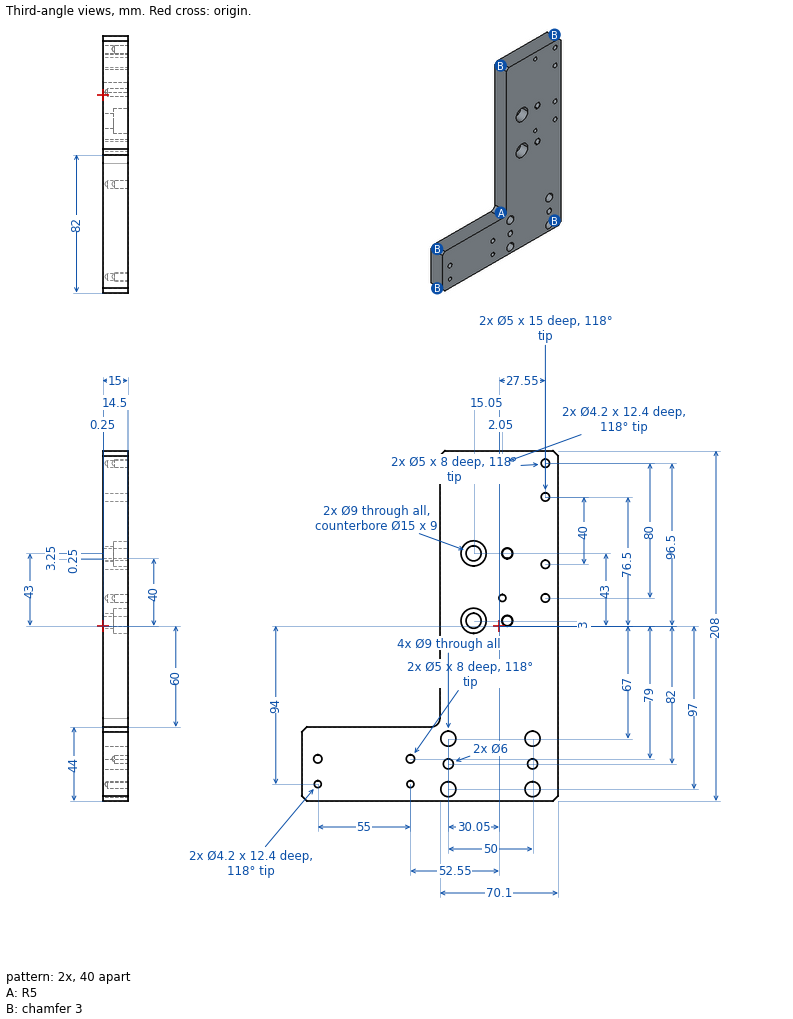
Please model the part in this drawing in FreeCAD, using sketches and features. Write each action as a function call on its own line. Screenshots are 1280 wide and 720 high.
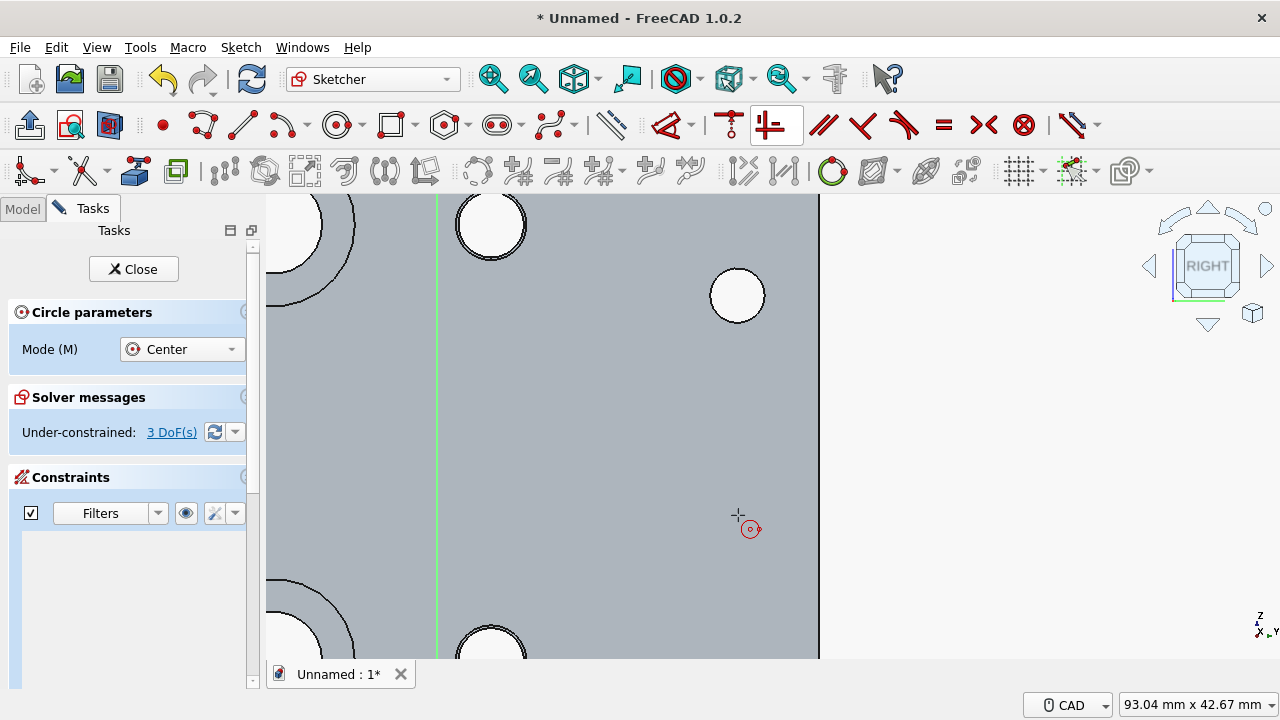
scroll(738, 516, down, 7)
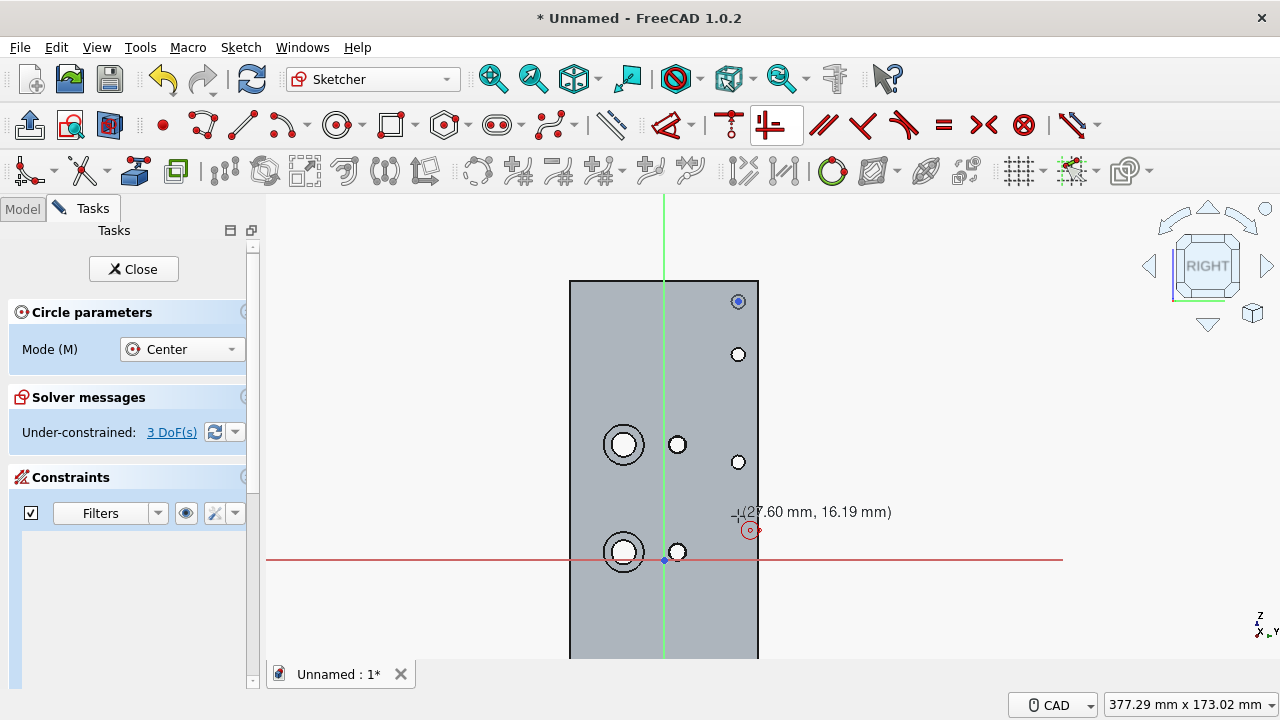
click(738, 516)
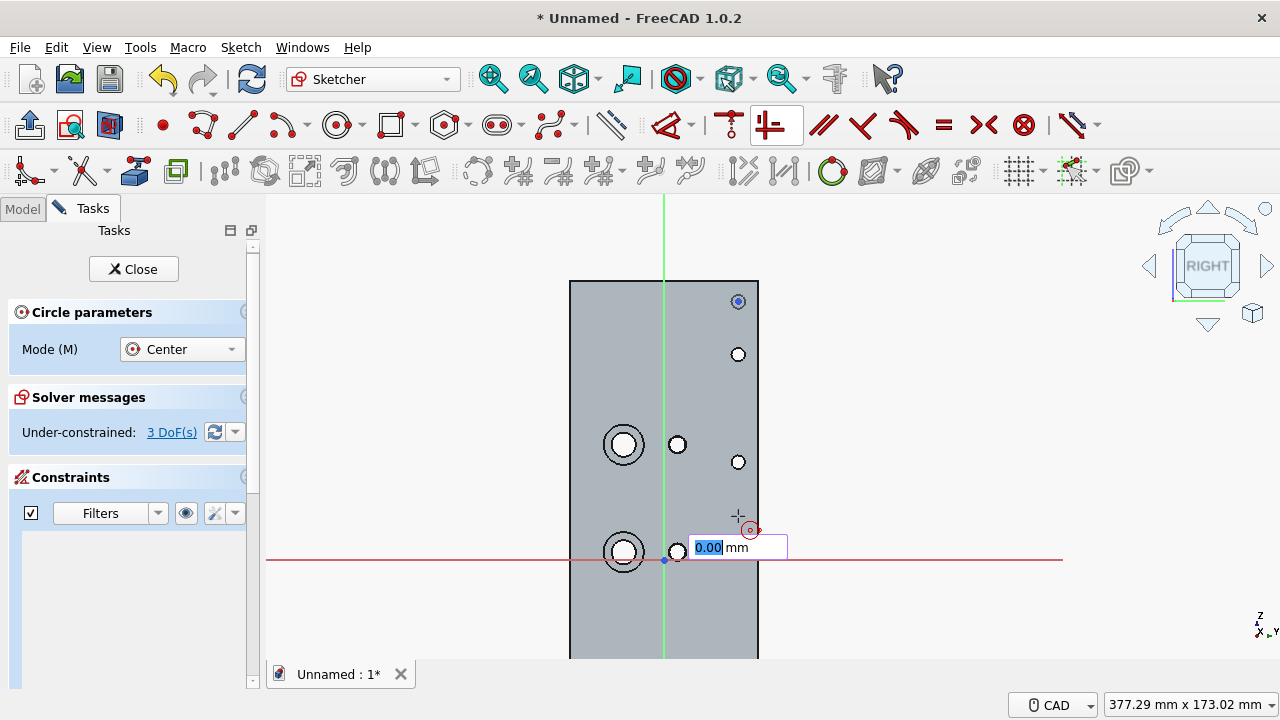
scroll(743, 511, up, 5)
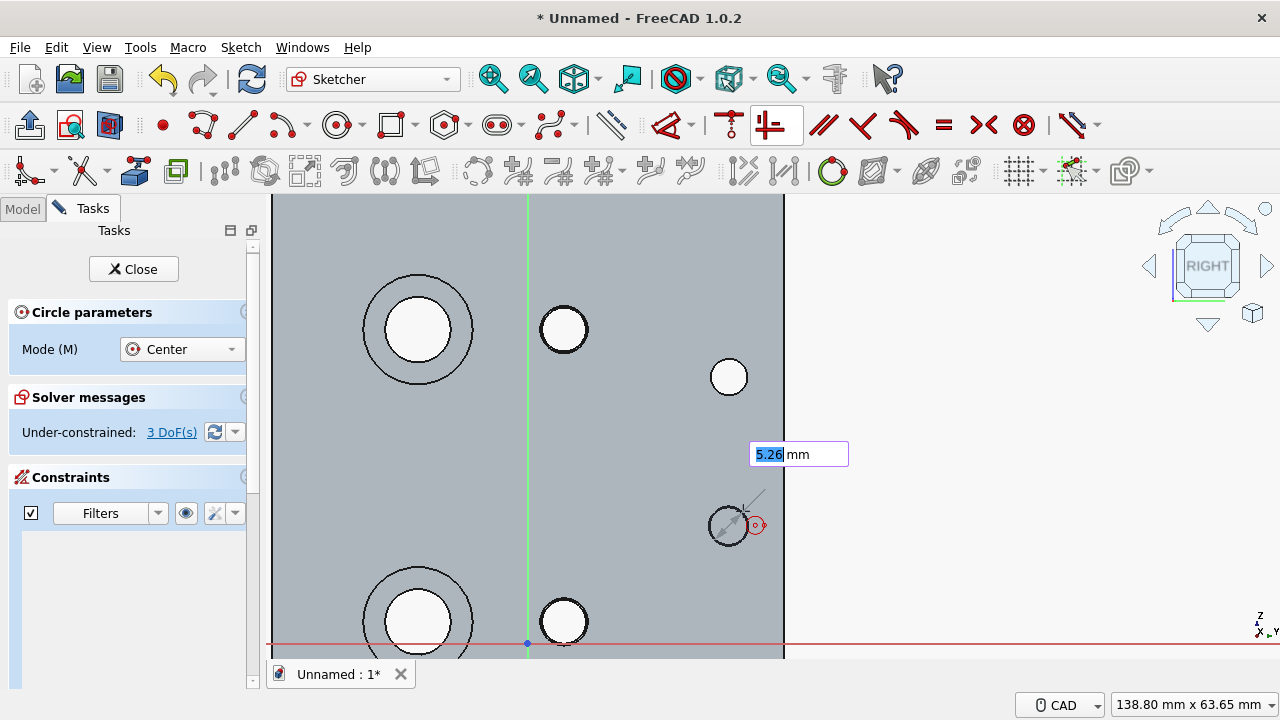
click(742, 510)
key(Escape)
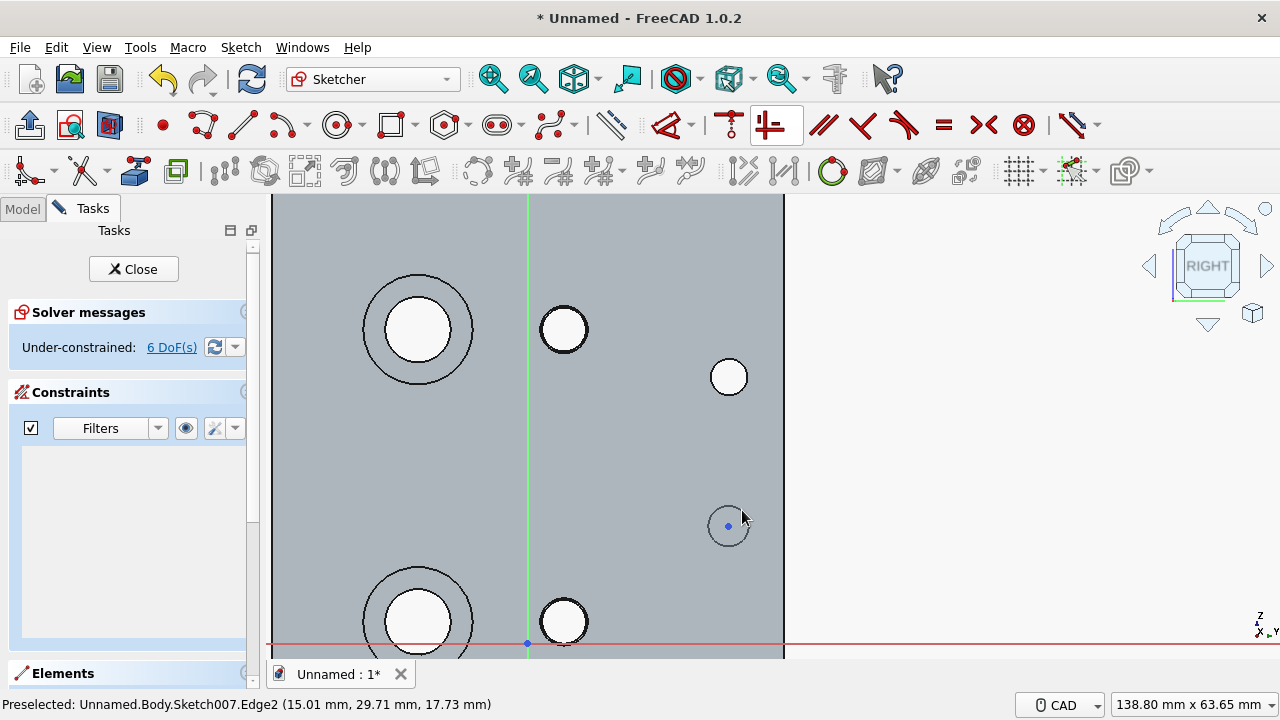
scroll(743, 511, down, 5)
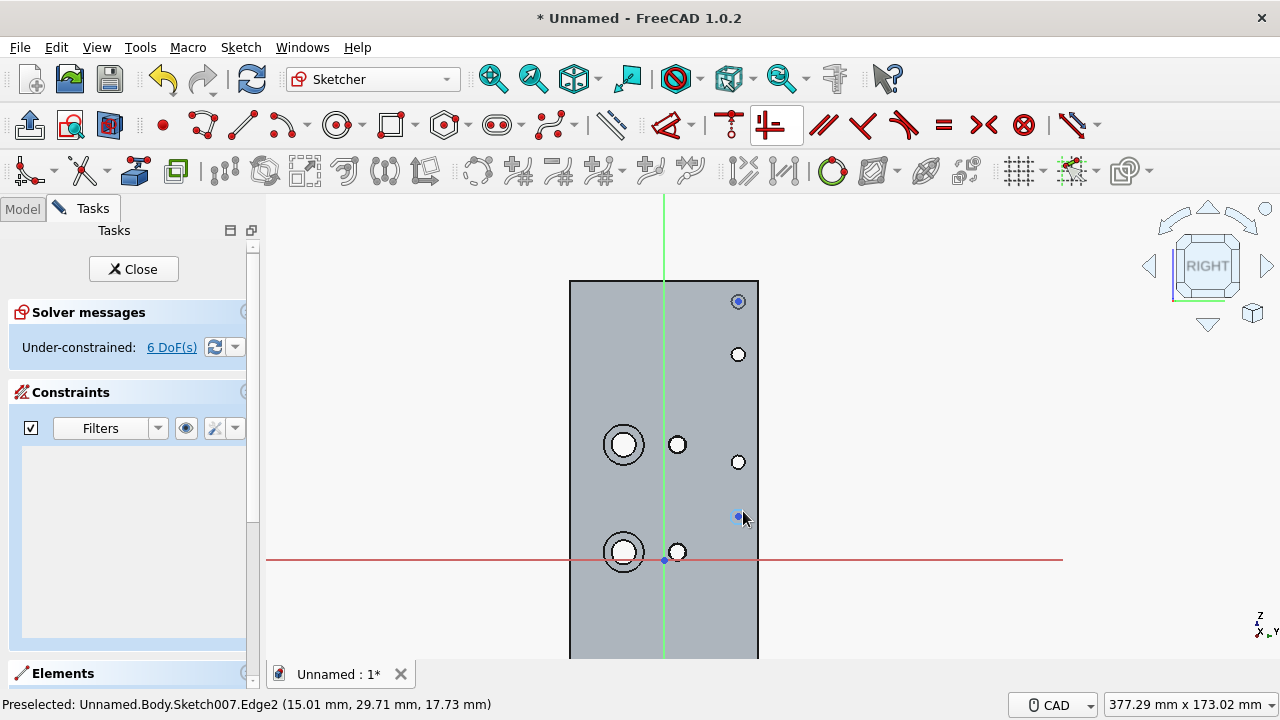
scroll(743, 297, up, 4)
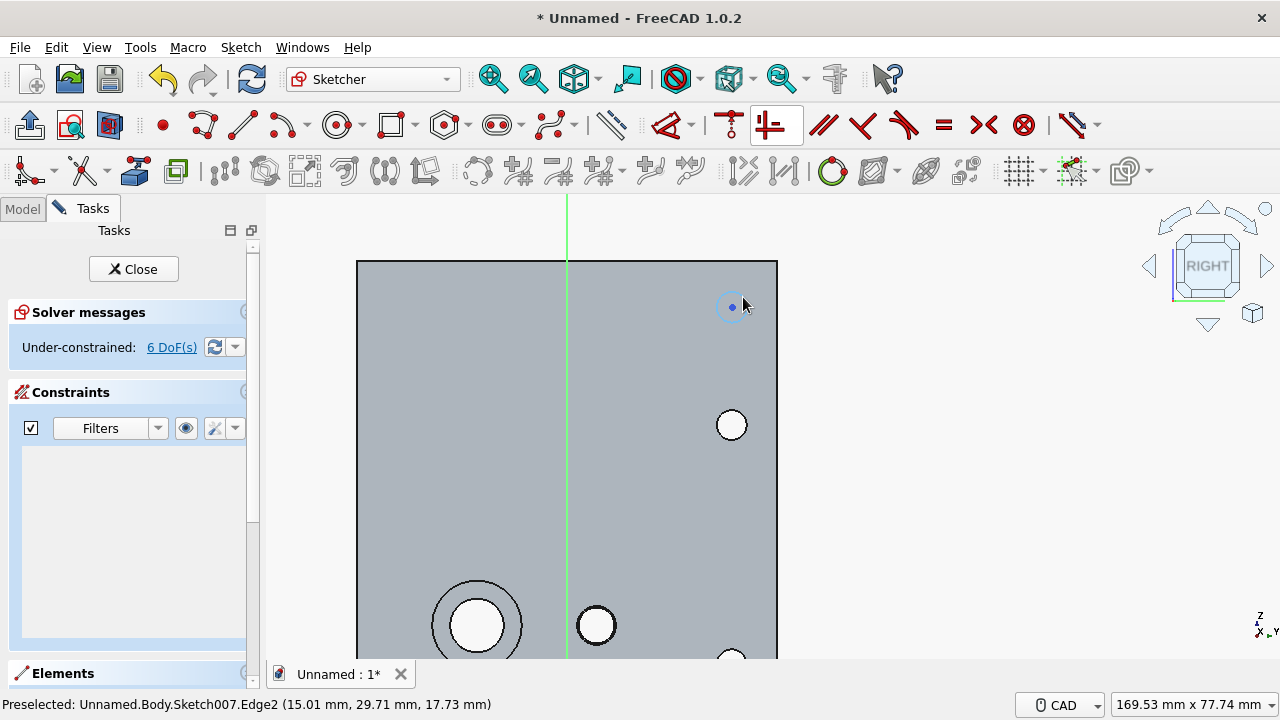
click(743, 296)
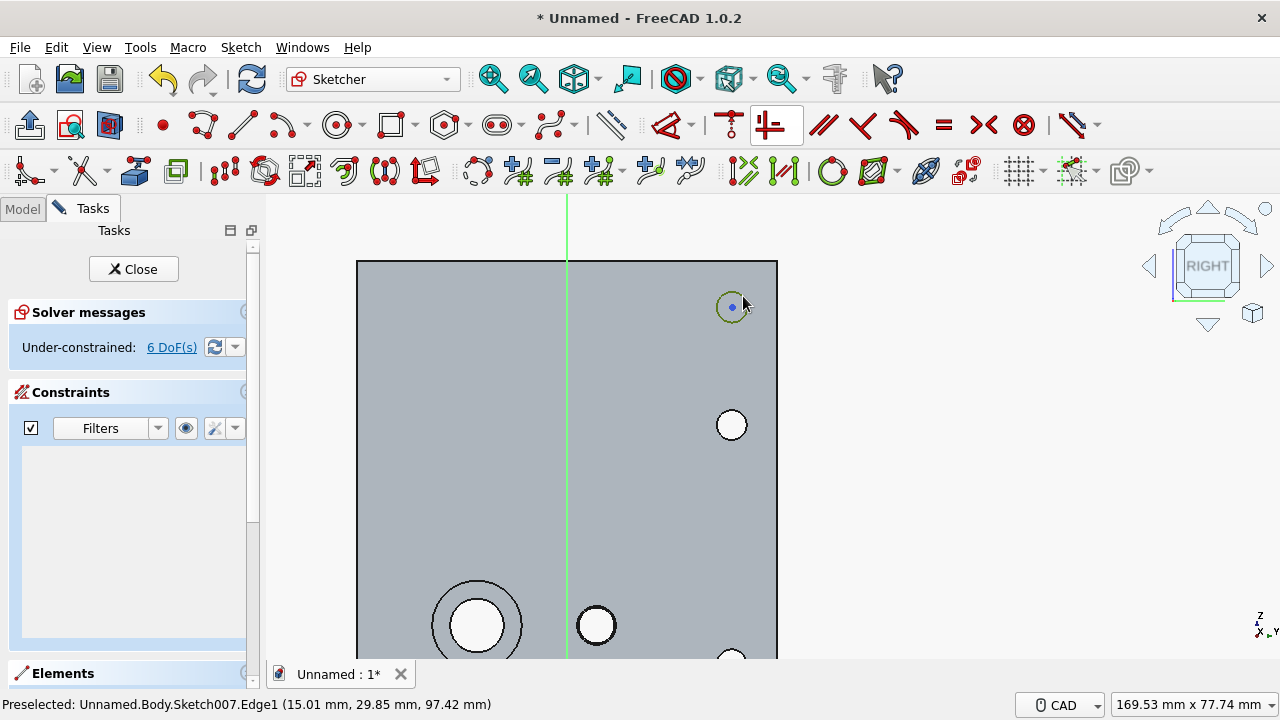
scroll(743, 296, down, 4)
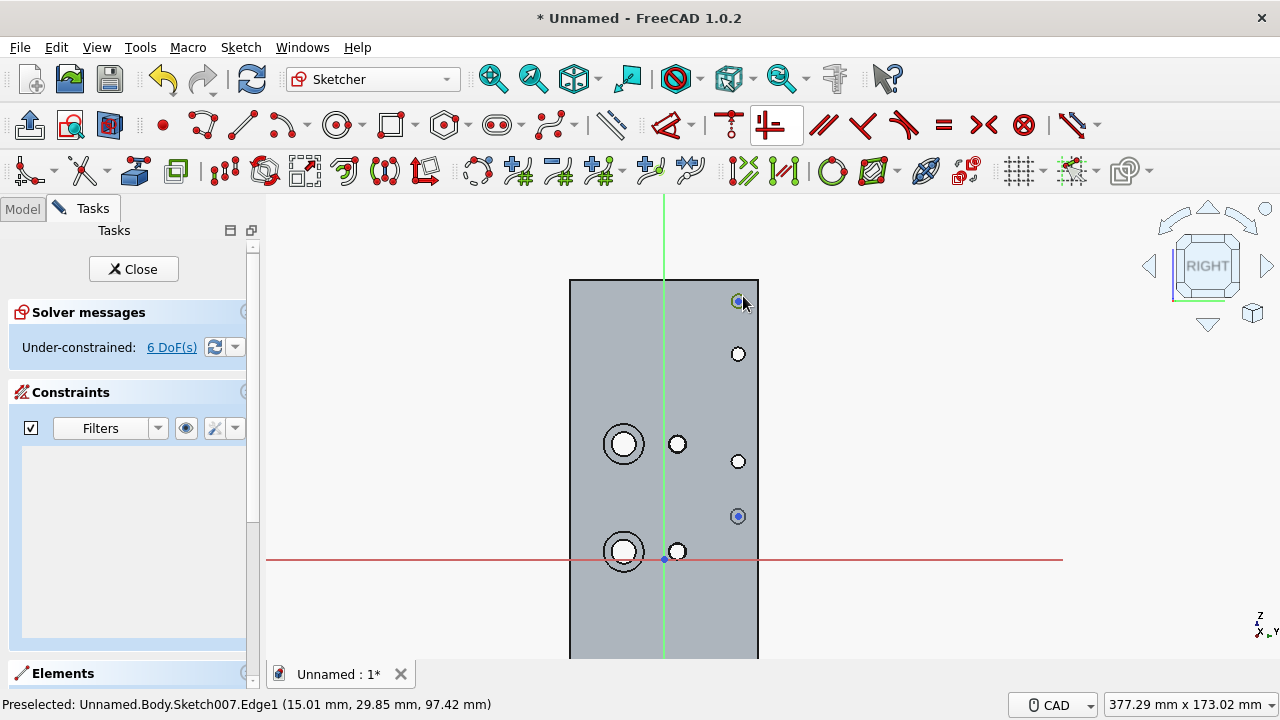
scroll(743, 511, up, 4)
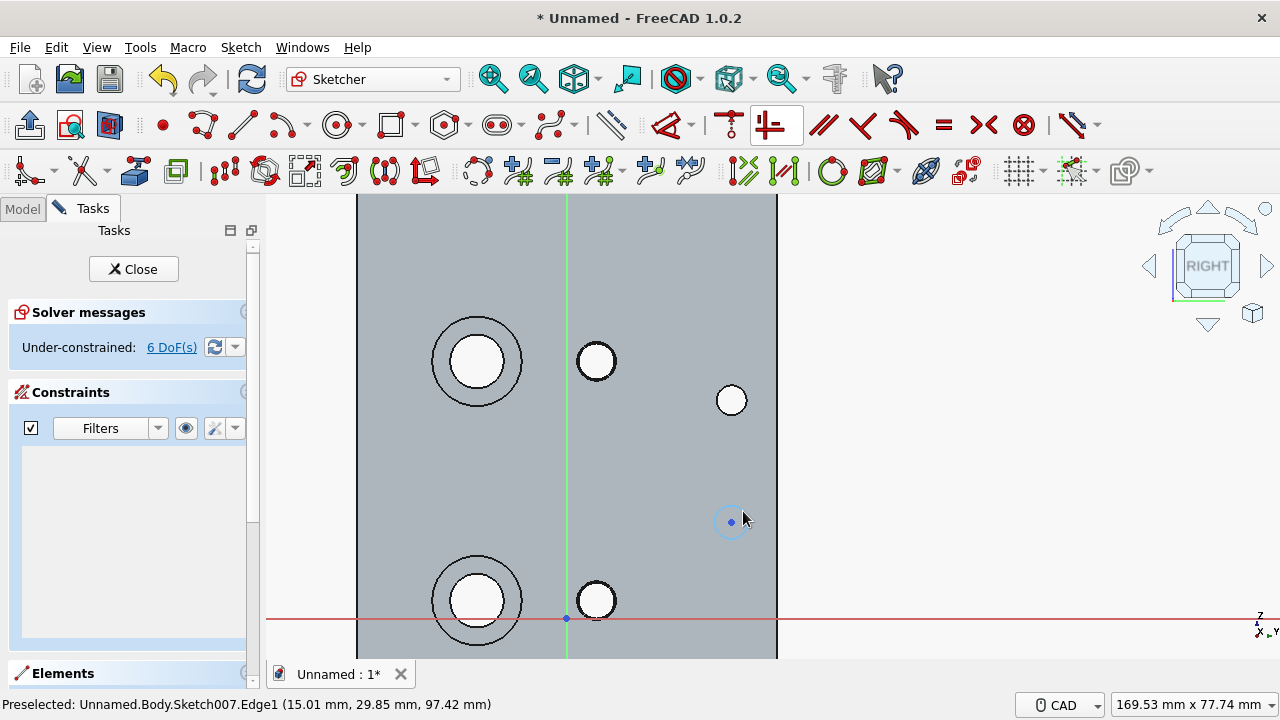
click(743, 511)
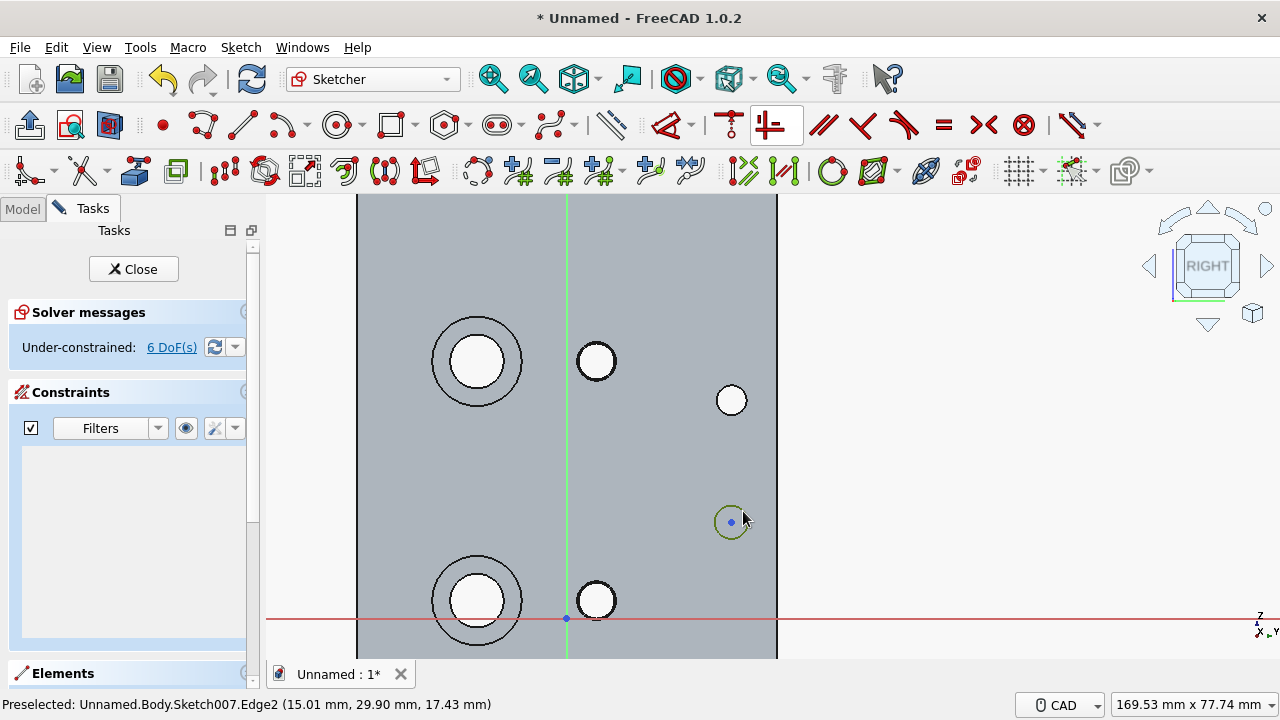
click(944, 126)